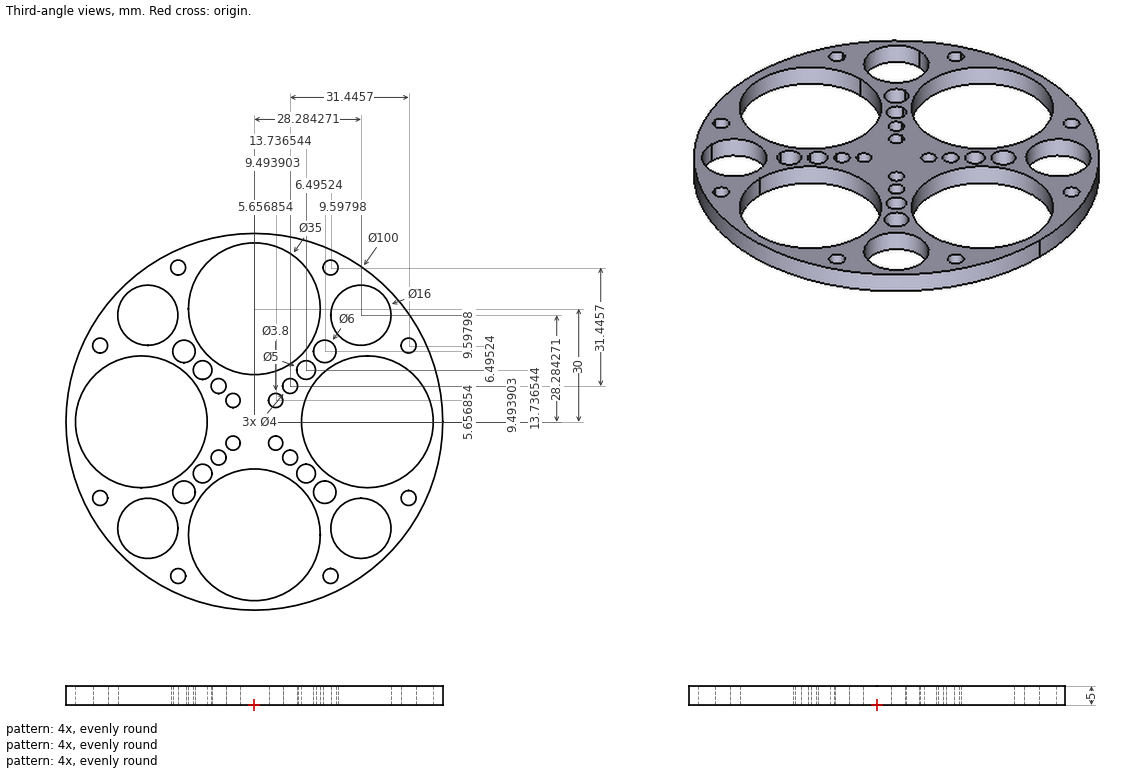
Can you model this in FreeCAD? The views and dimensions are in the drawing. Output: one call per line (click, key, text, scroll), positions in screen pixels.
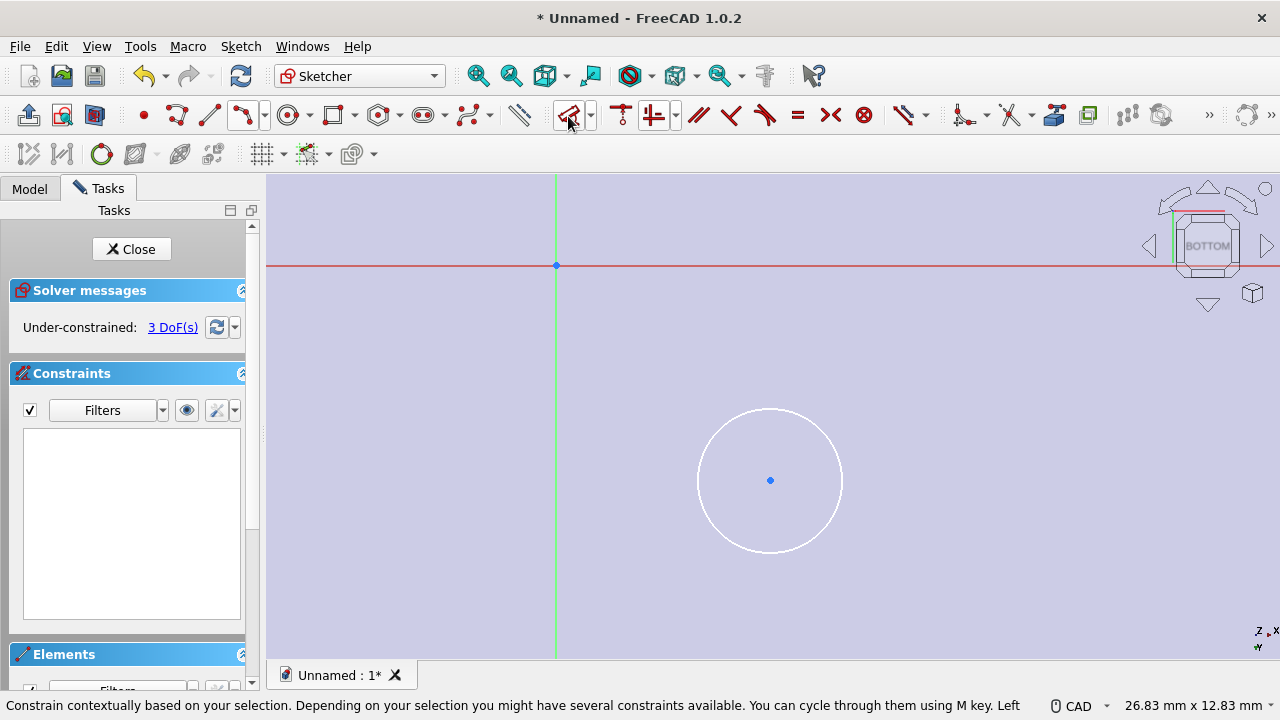
click(821, 430)
click(844, 407)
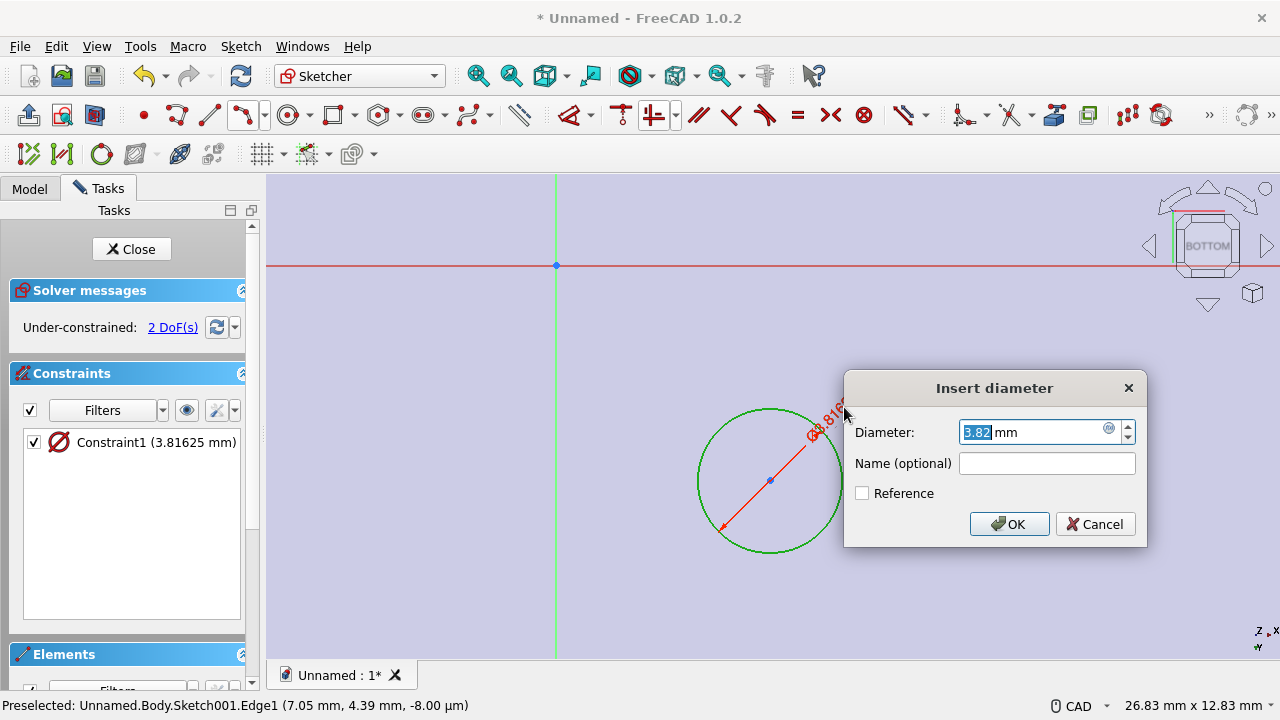
text(3.8)
key(Return)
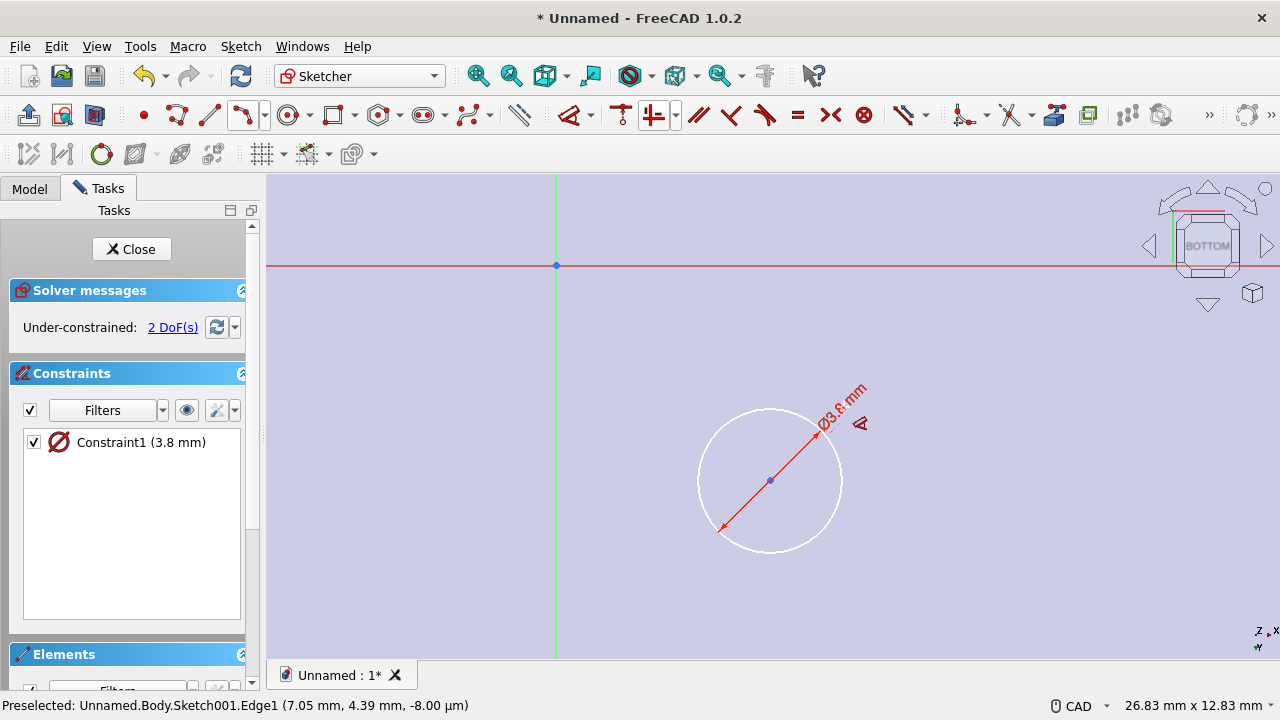
click(770, 481)
click(663, 232)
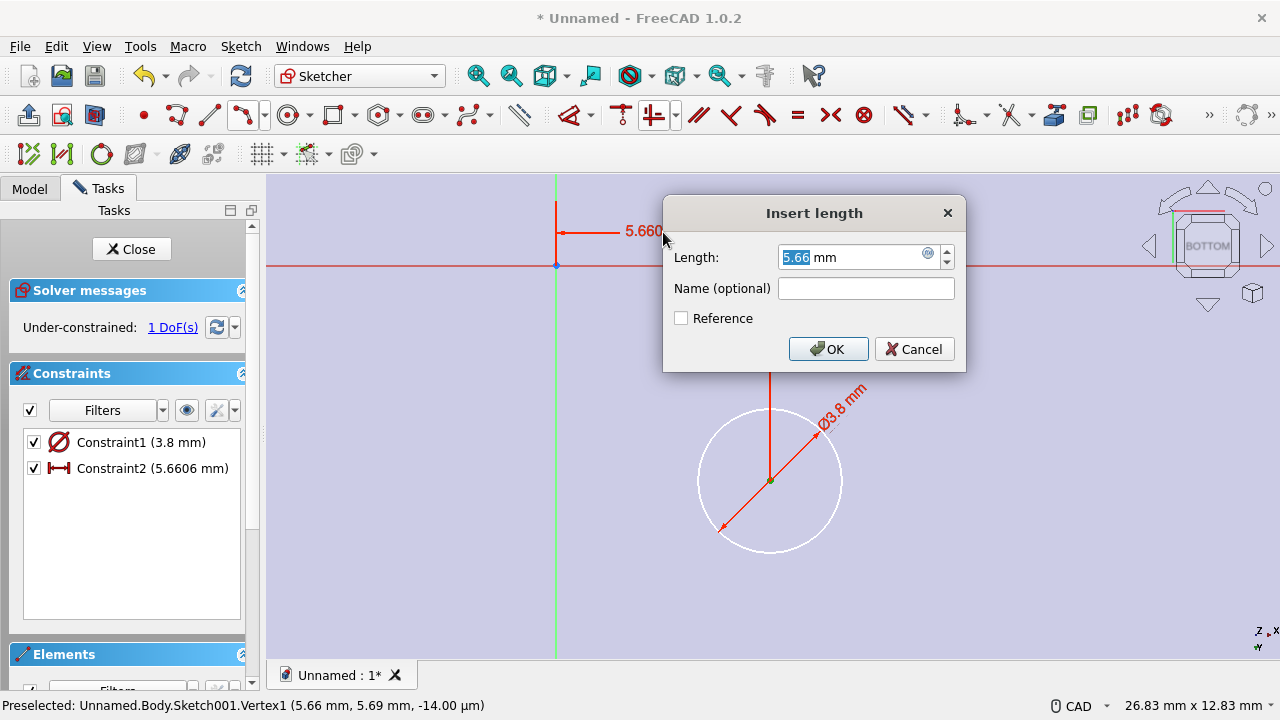
text(5.656854)
key(Return)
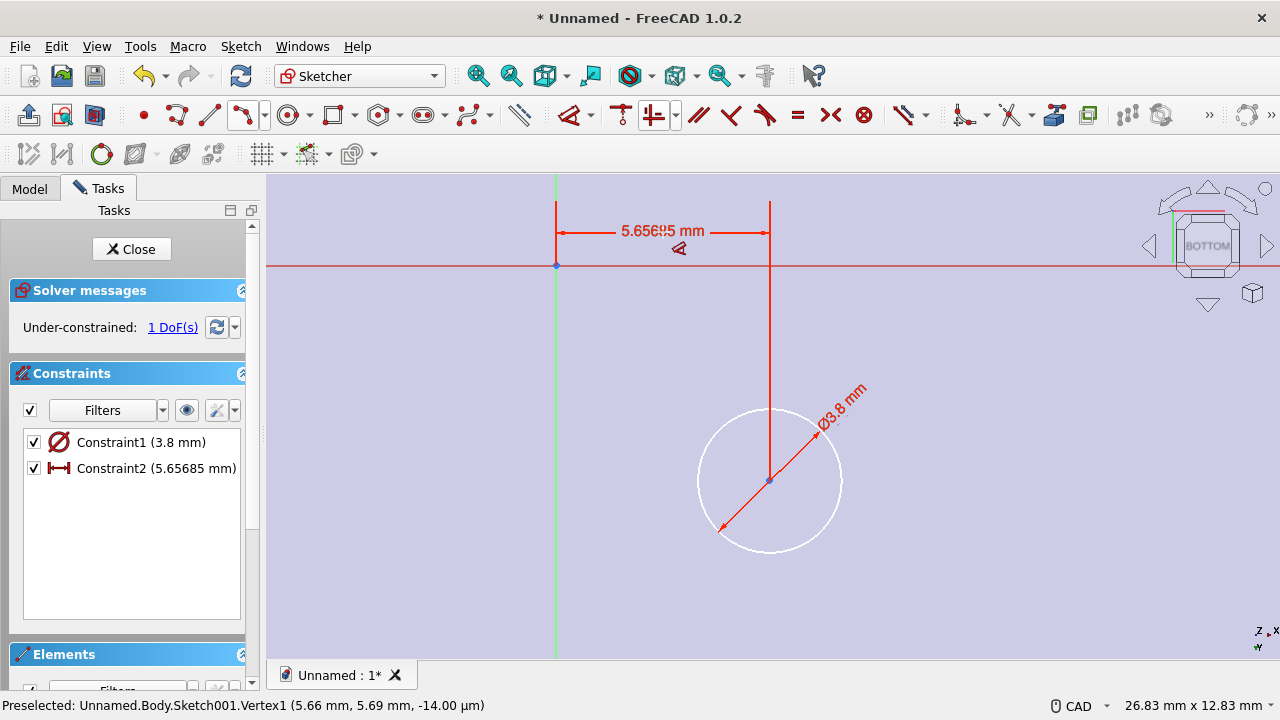
click(770, 481)
click(522, 373)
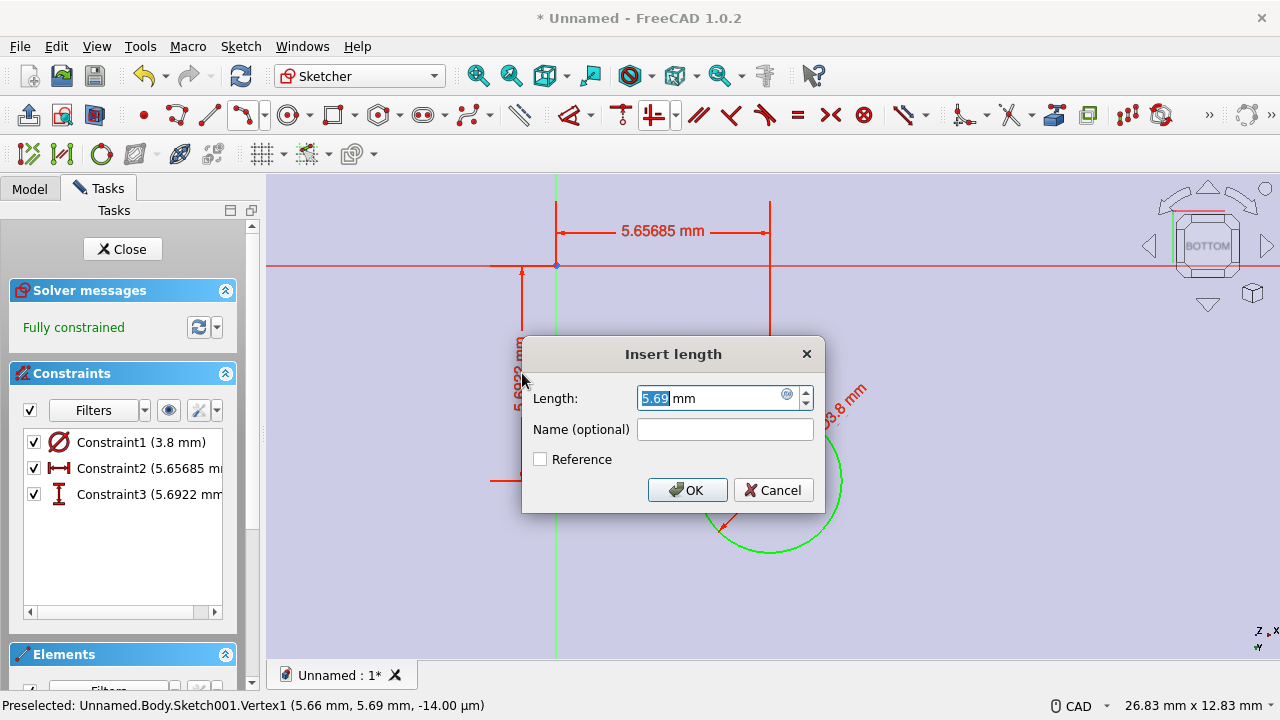
text(5.656854)
key(Return)
key(Escape)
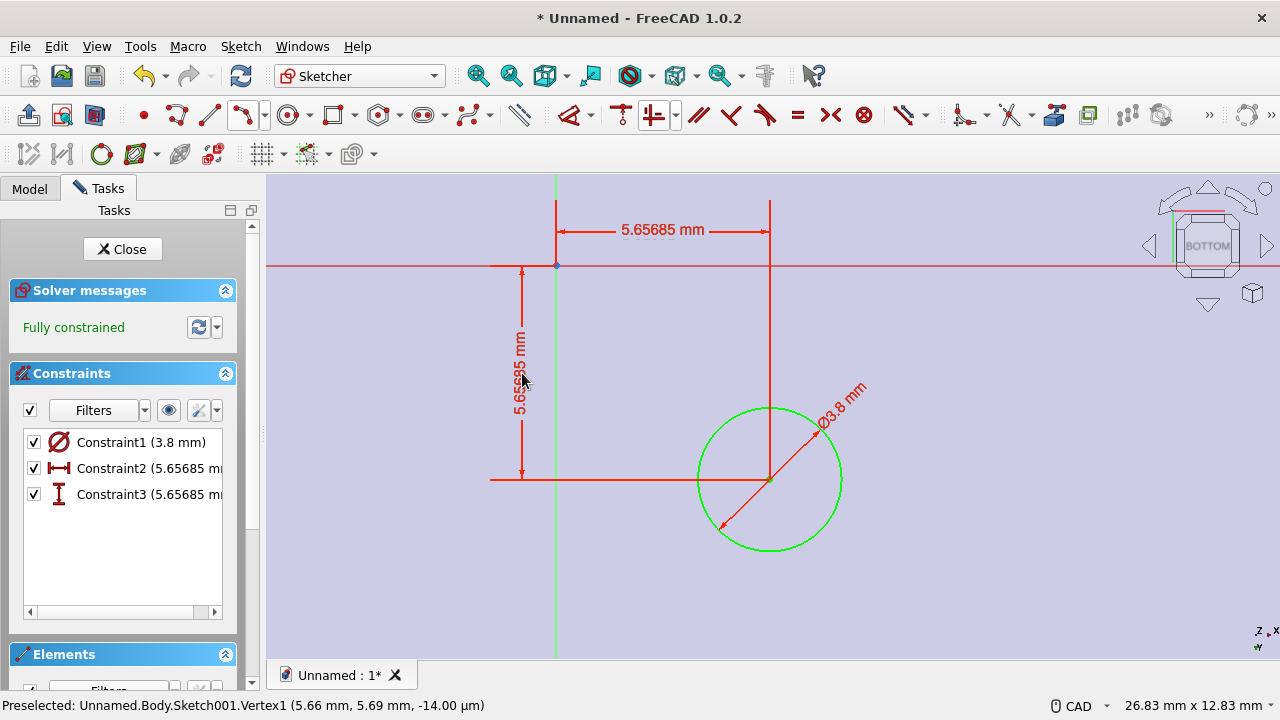
click(123, 249)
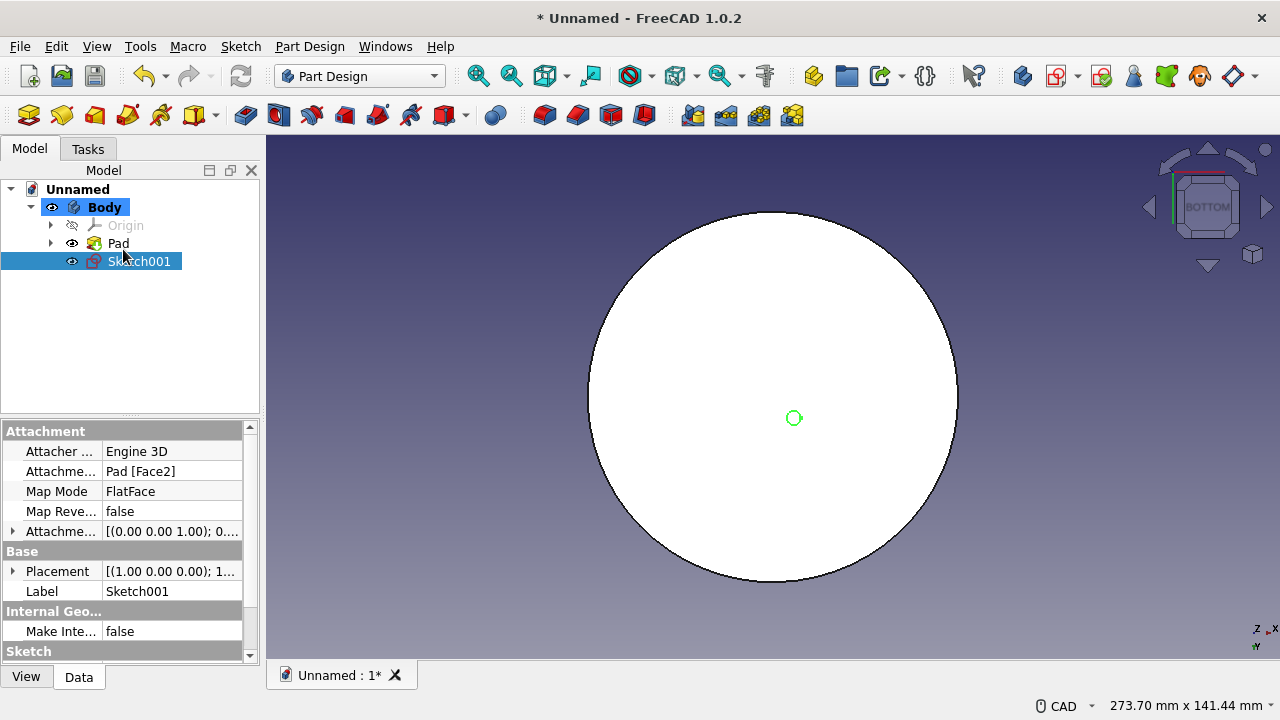
click(246, 116)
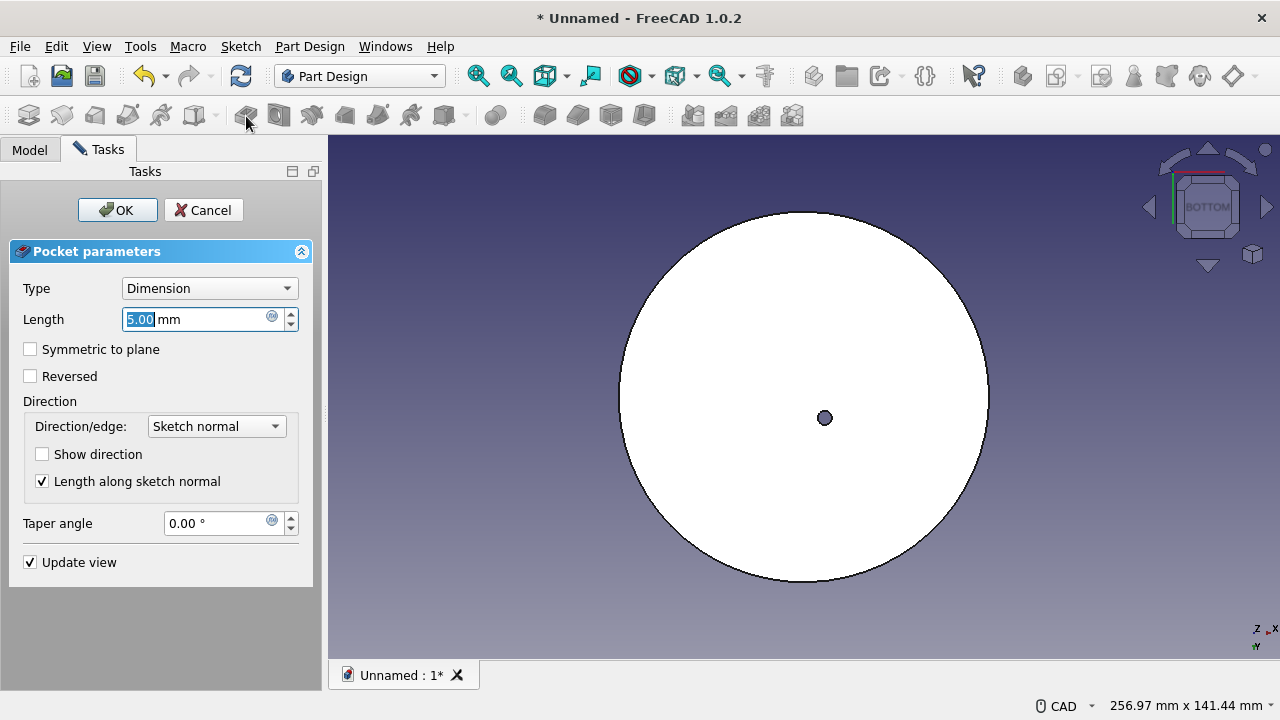
click(210, 288)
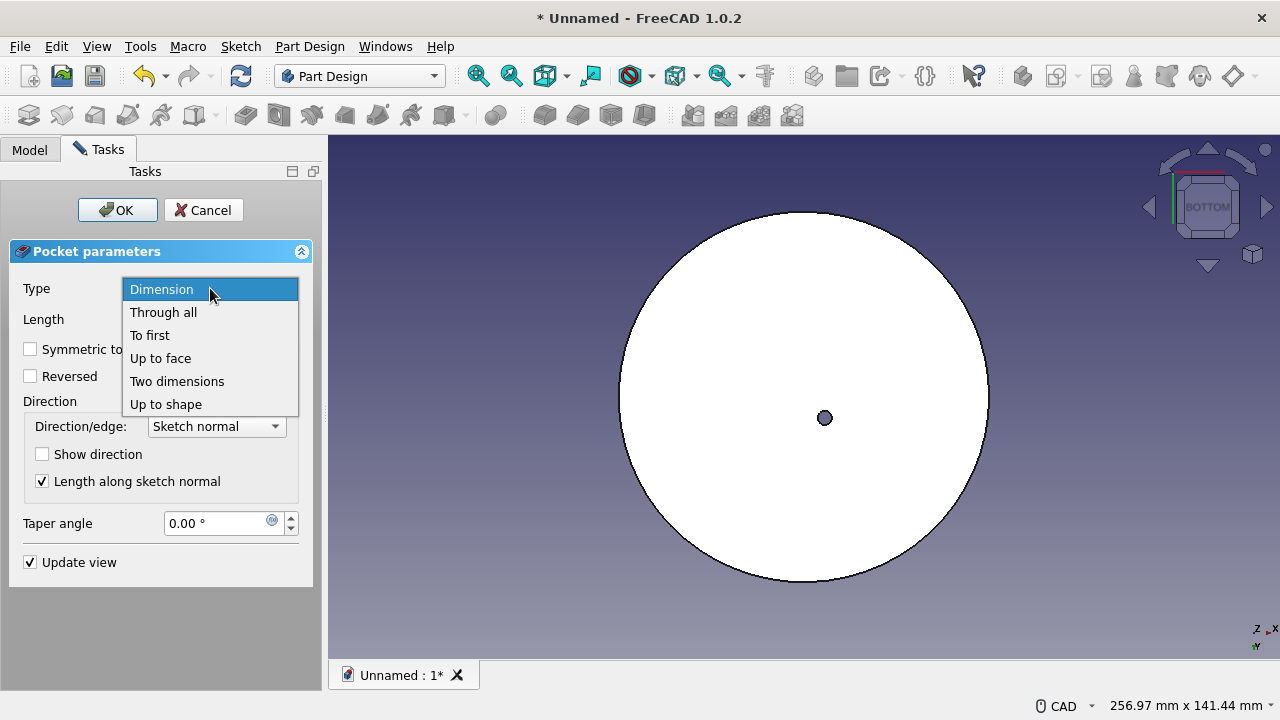
click(208, 312)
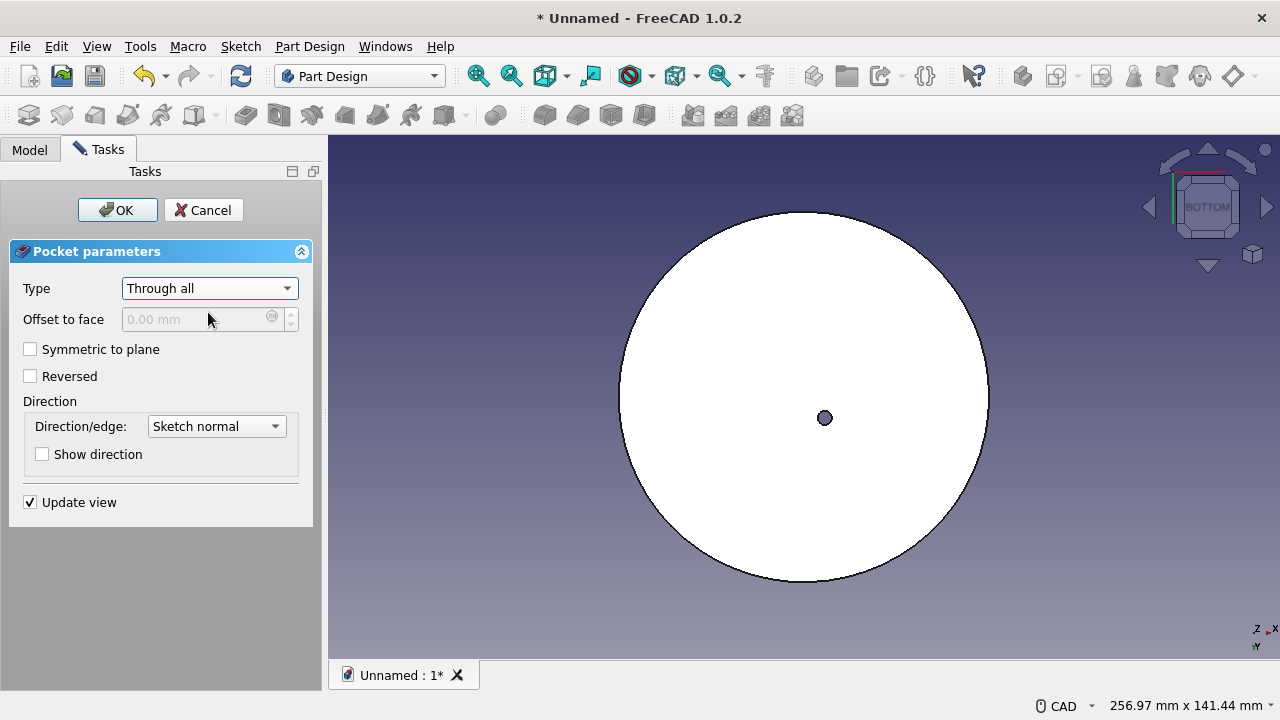
click(118, 210)